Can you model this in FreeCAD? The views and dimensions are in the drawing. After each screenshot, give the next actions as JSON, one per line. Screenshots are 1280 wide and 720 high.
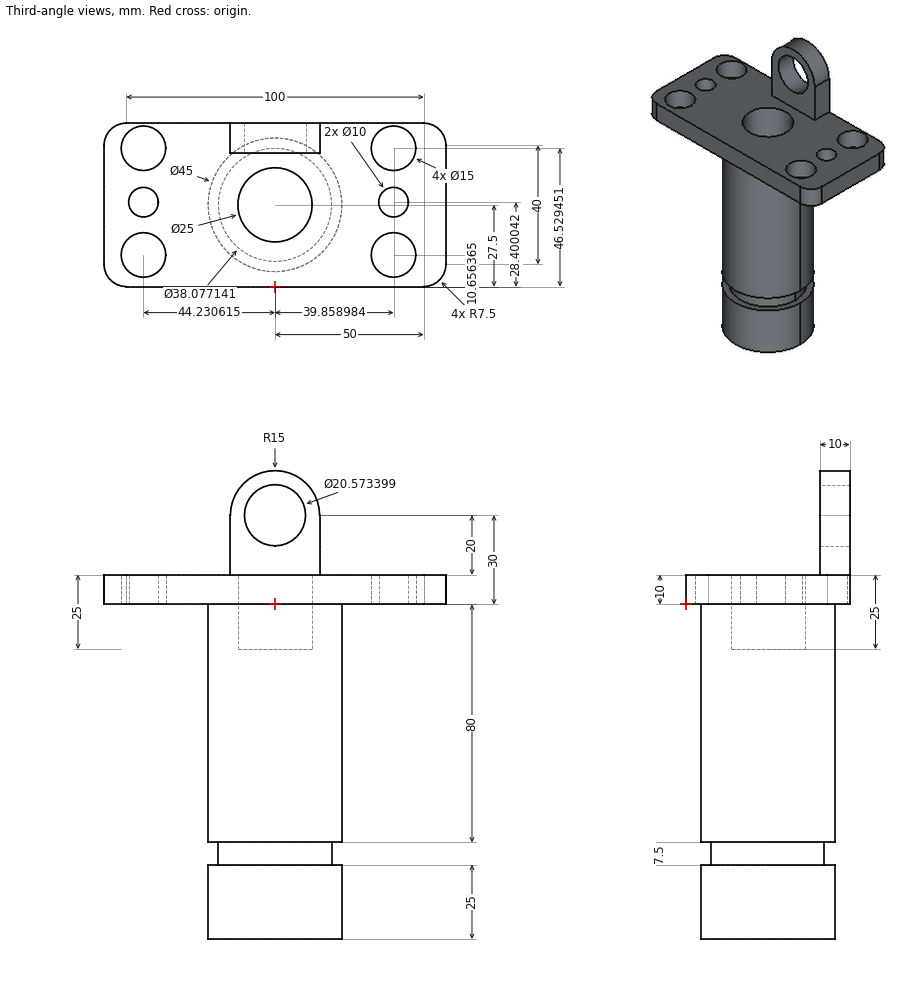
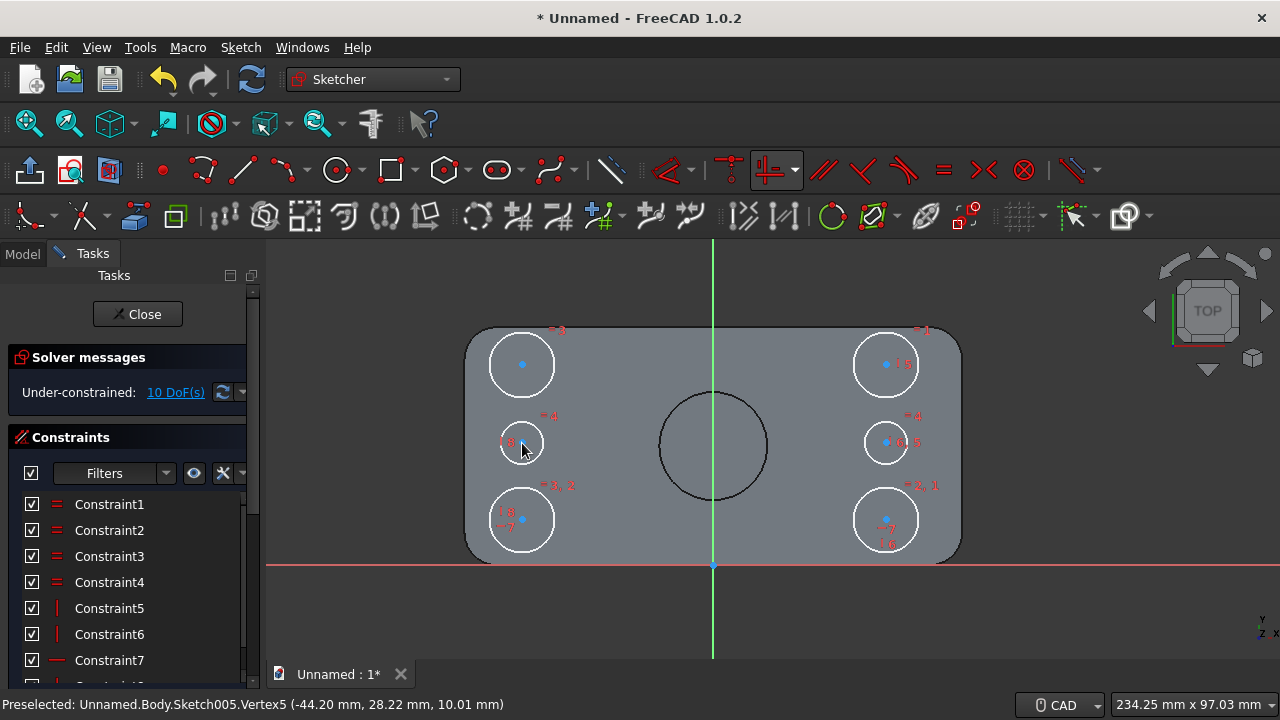
{"action": "left_click", "coordinate": [886, 443]}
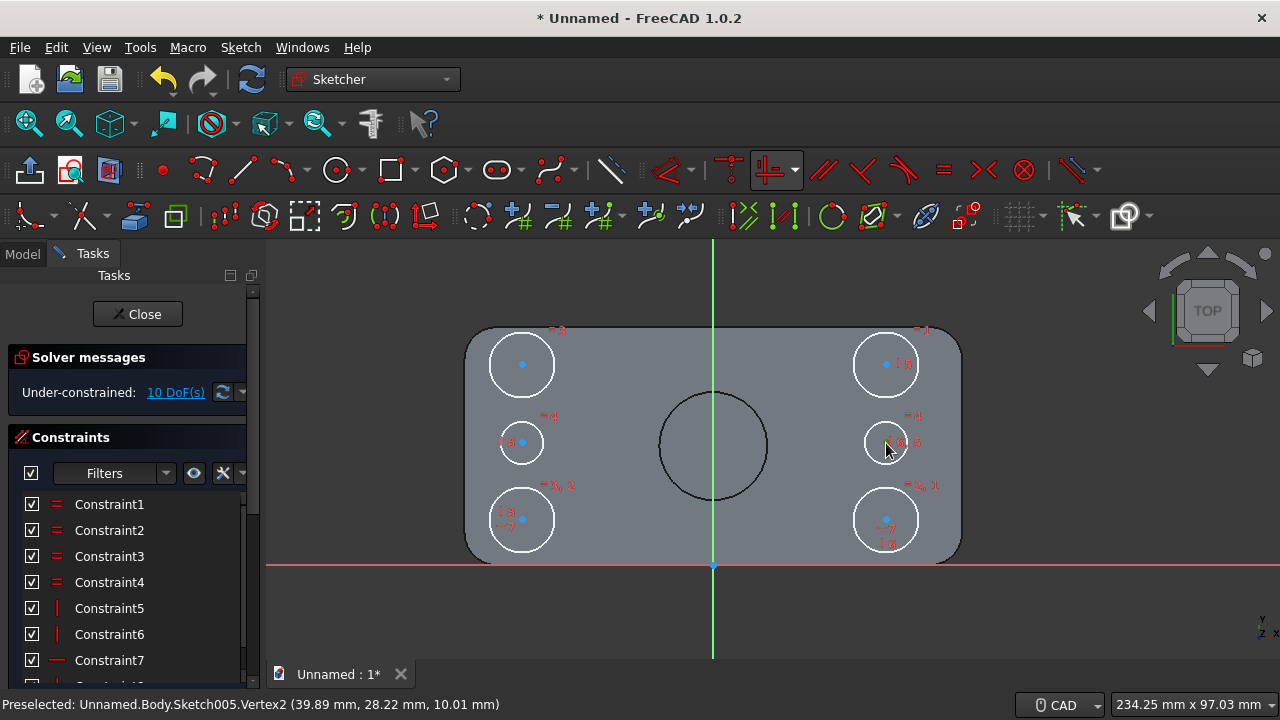
{"action": "left_click", "coordinate": [522, 443]}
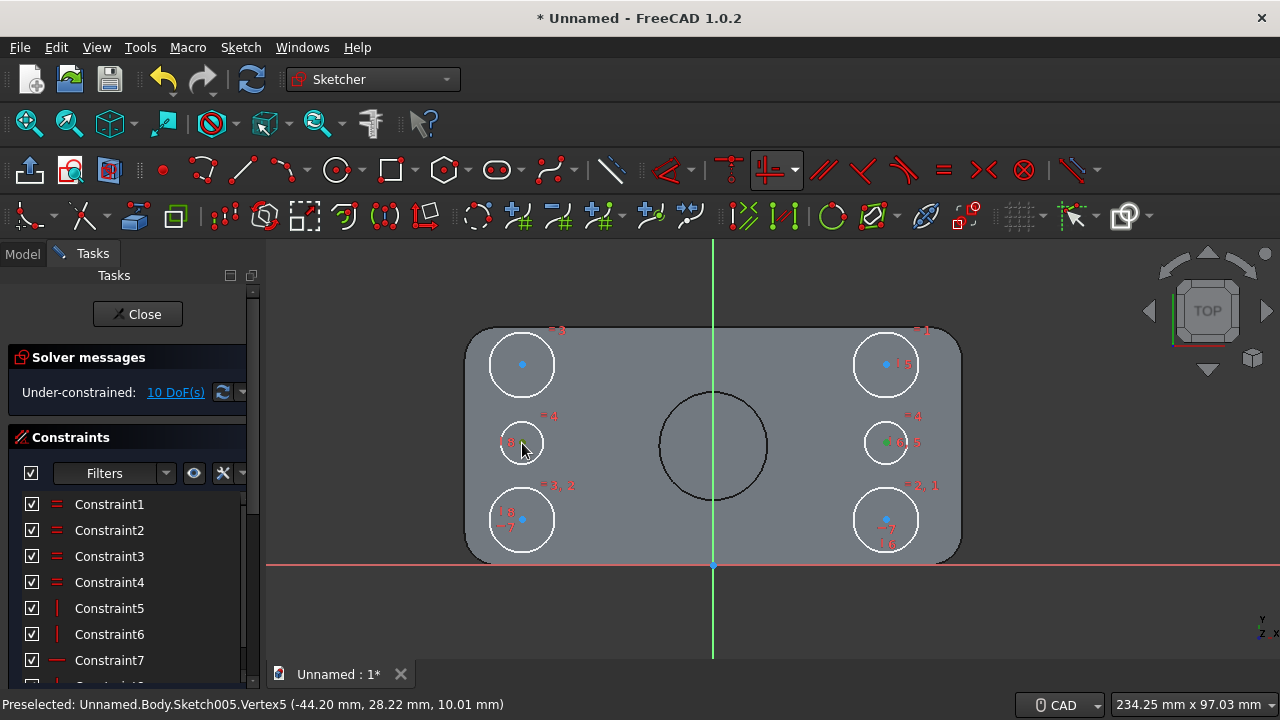
{"action": "key", "text": "h"}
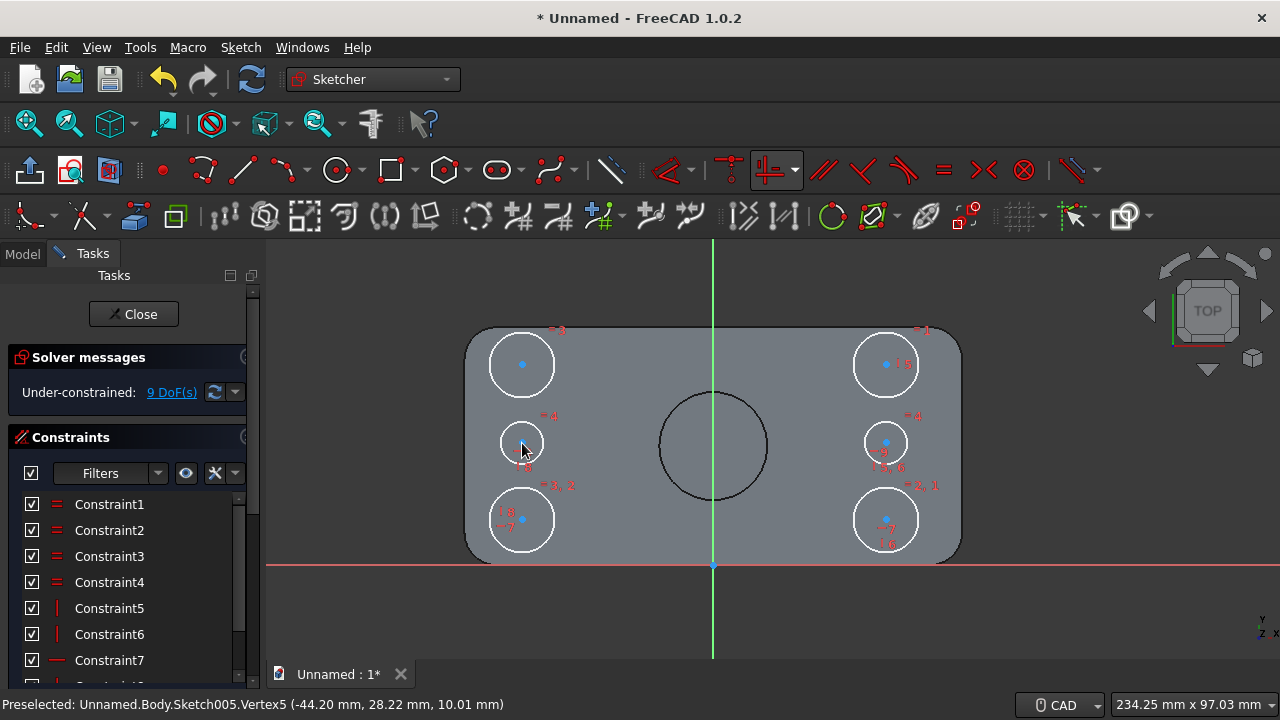
{"action": "left_click", "coordinate": [522, 443]}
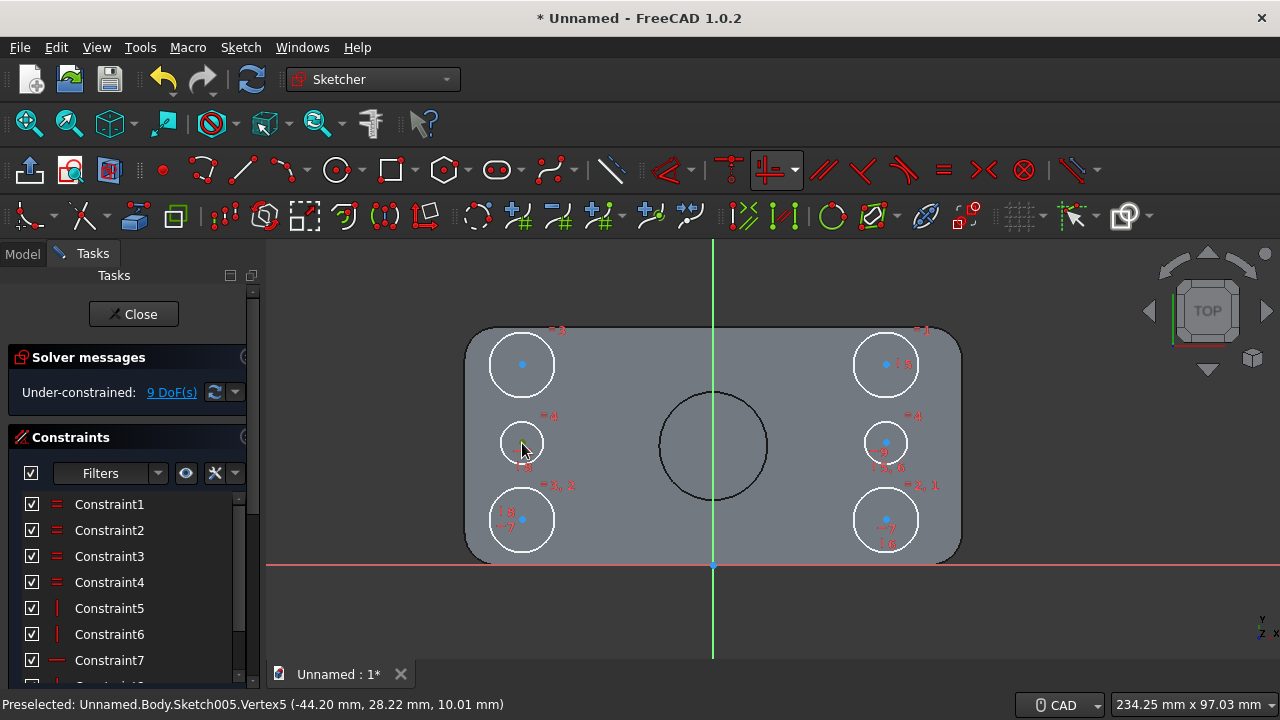
{"action": "left_click", "coordinate": [522, 365]}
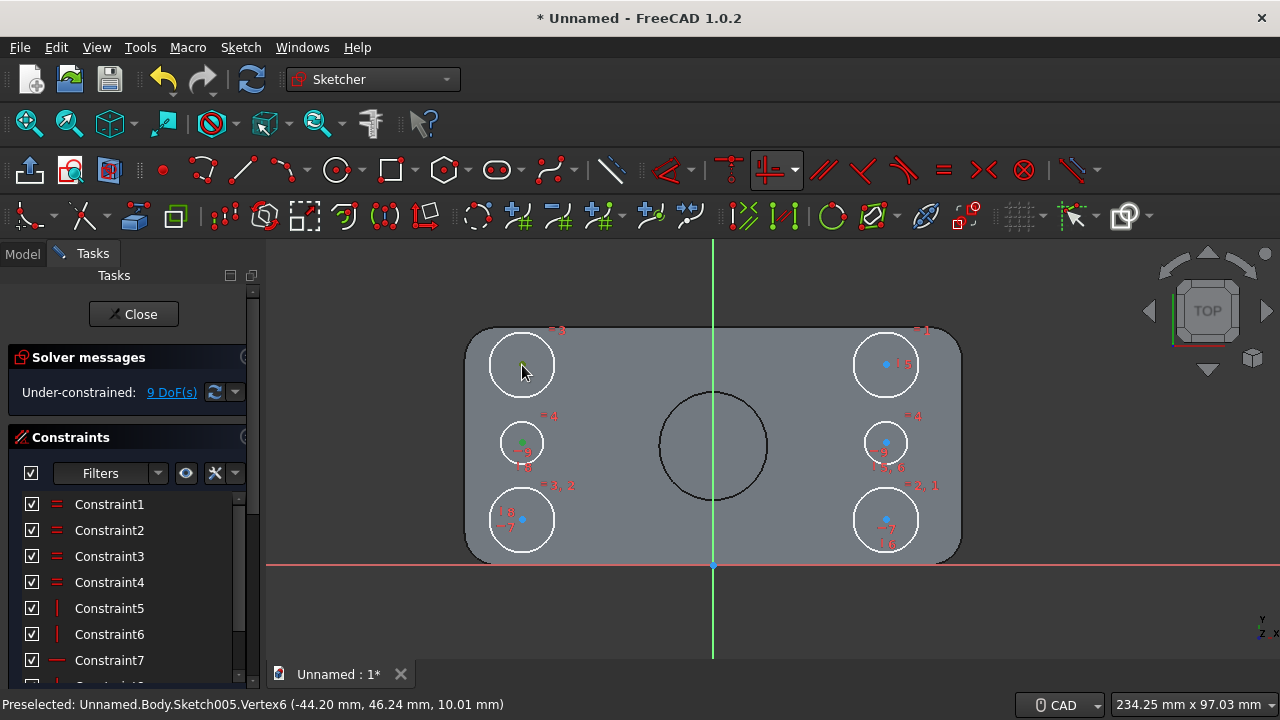
{"action": "left_click", "coordinate": [798, 170]}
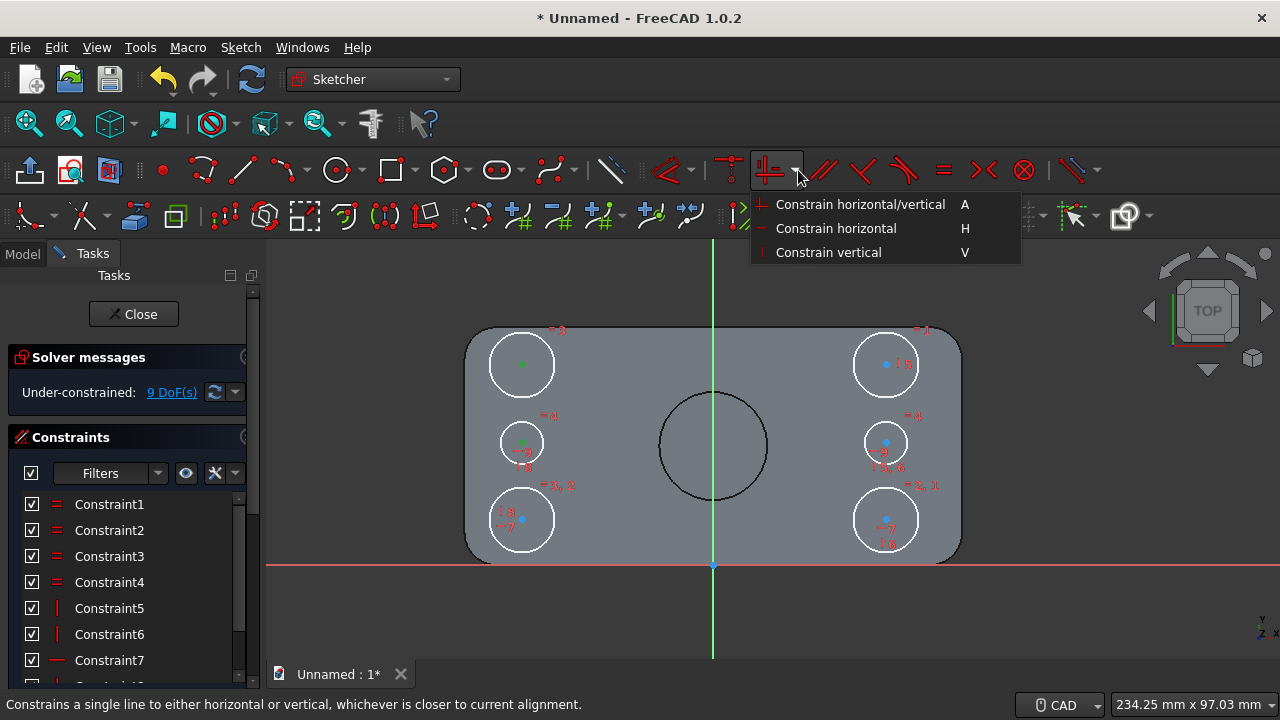
{"action": "left_click", "coordinate": [886, 252]}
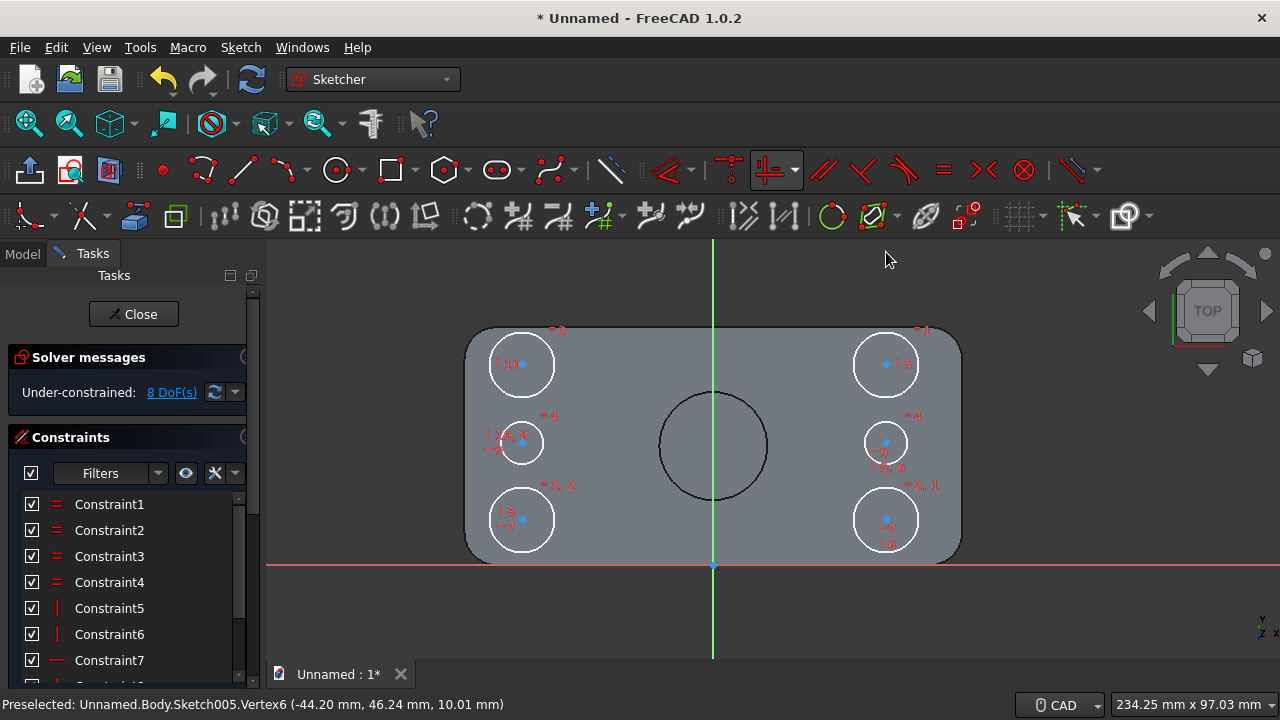
{"action": "left_click", "coordinate": [886, 365]}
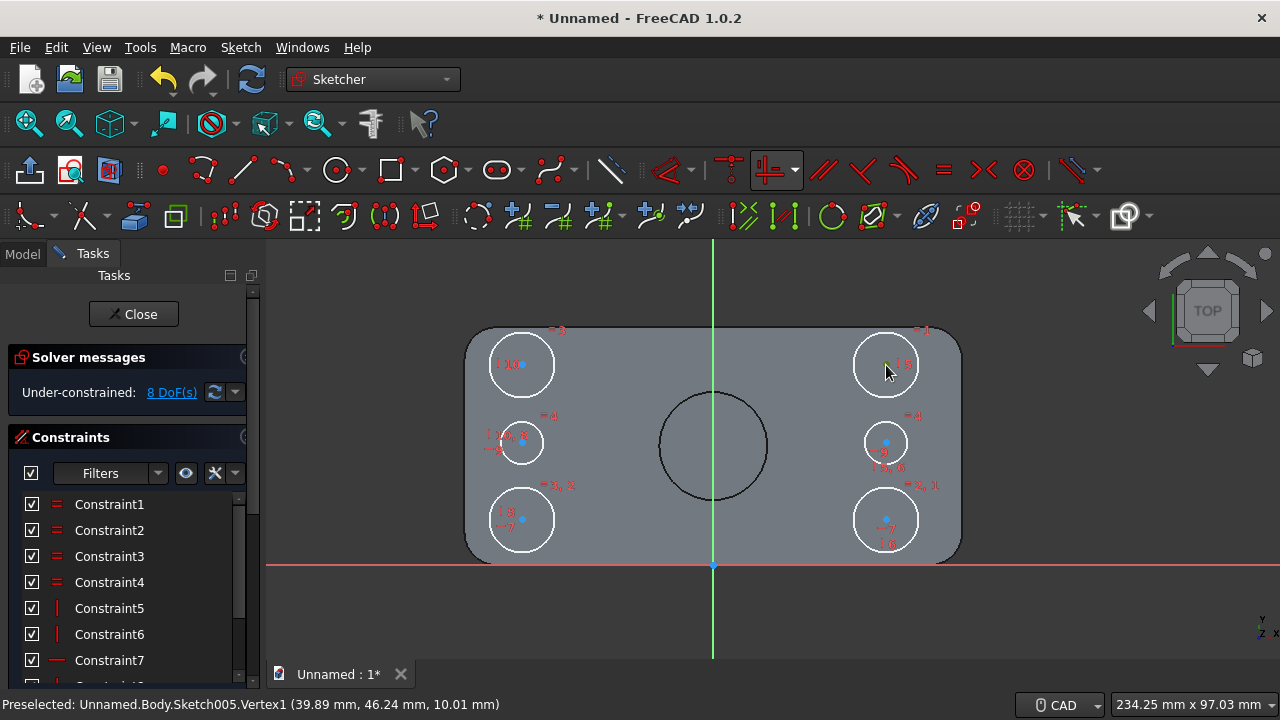
{"action": "left_click", "coordinate": [522, 365]}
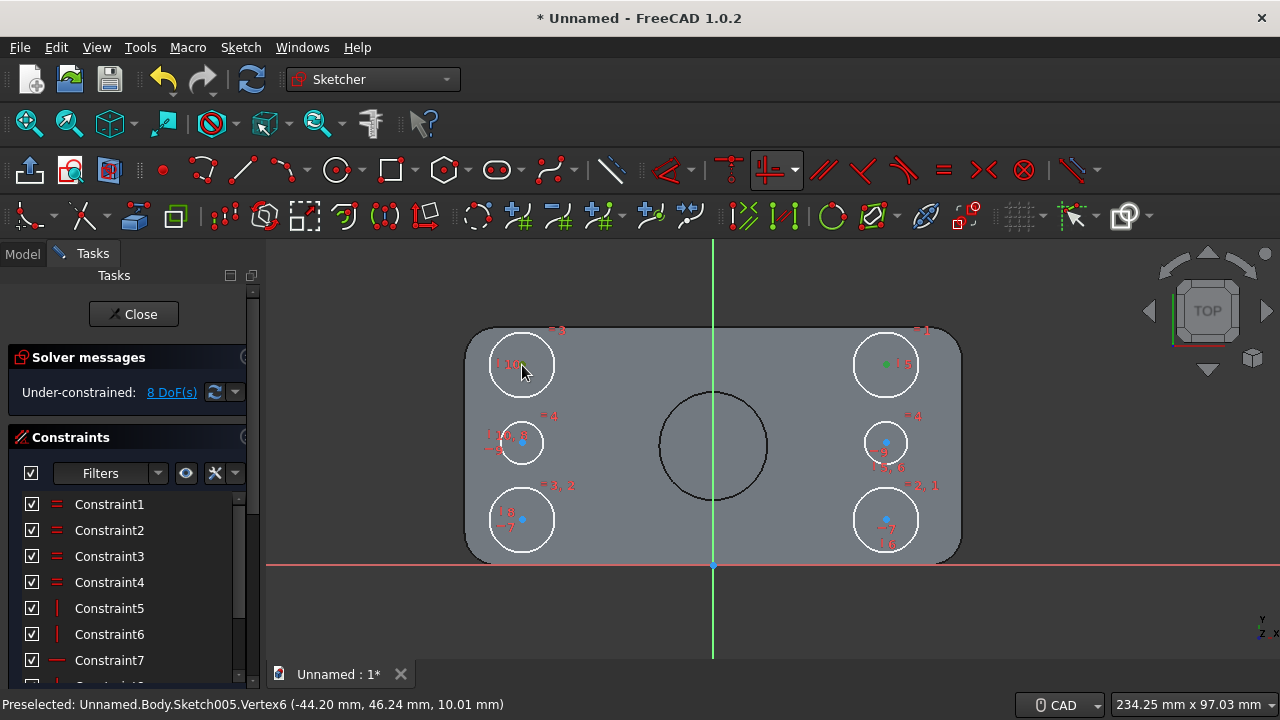
{"action": "left_click", "coordinate": [798, 170]}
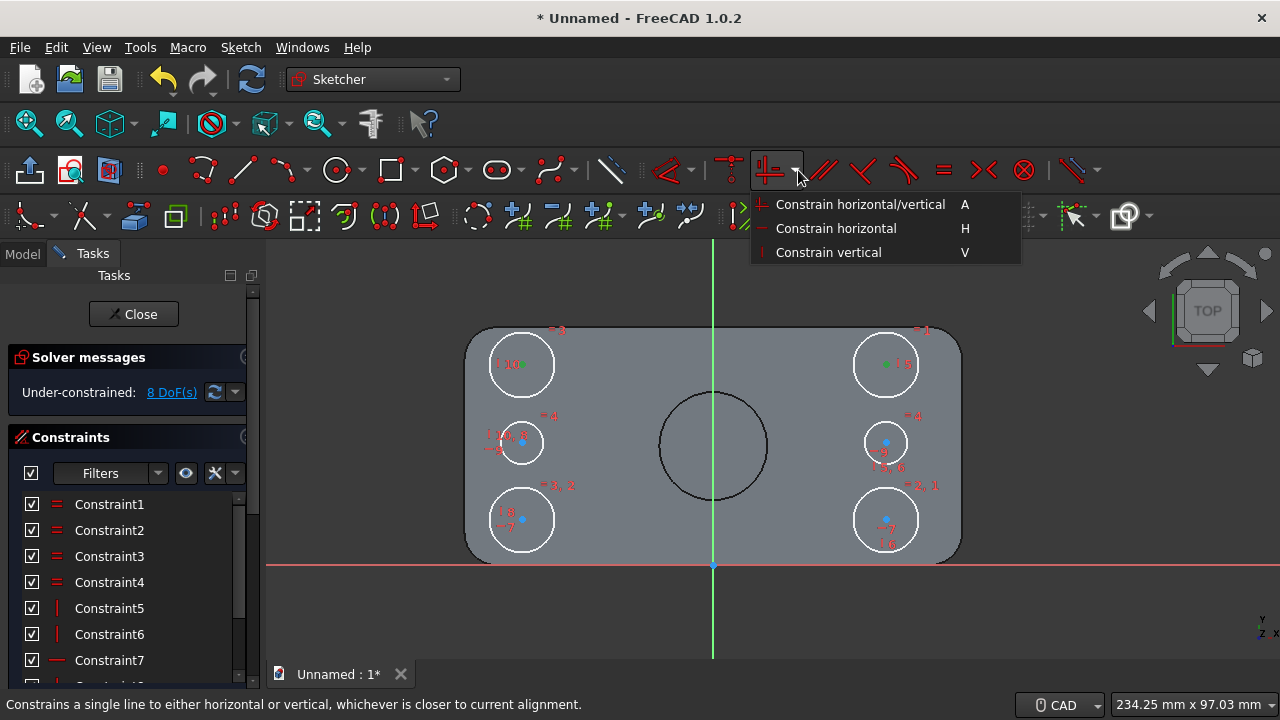
{"action": "left_click", "coordinate": [886, 228]}